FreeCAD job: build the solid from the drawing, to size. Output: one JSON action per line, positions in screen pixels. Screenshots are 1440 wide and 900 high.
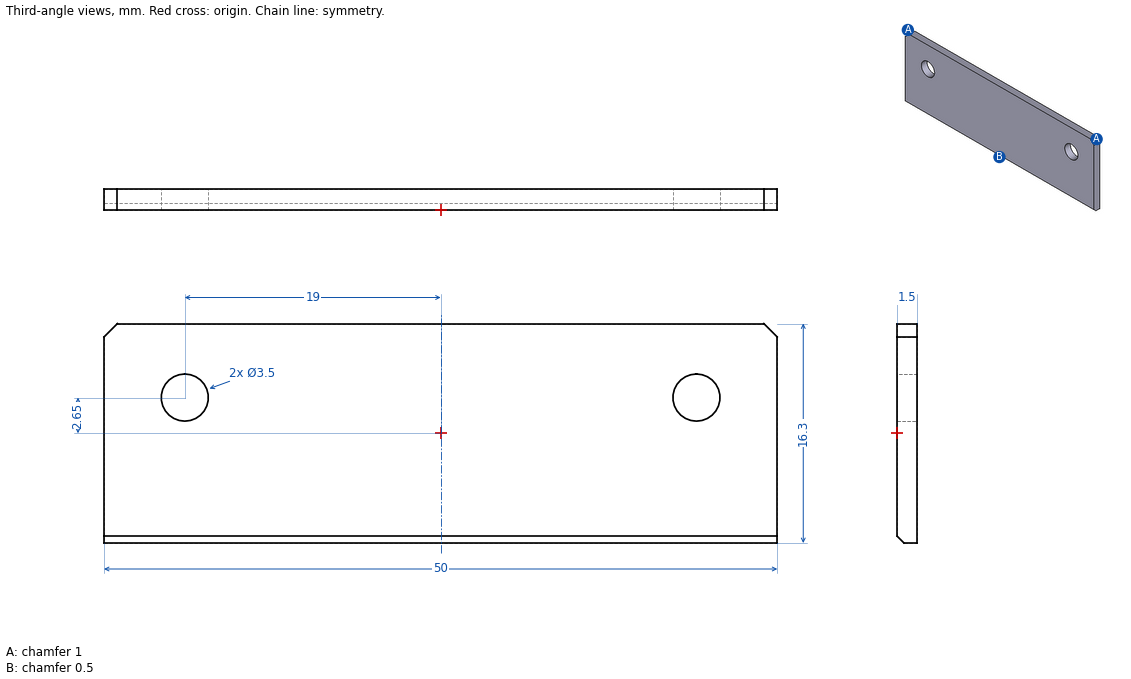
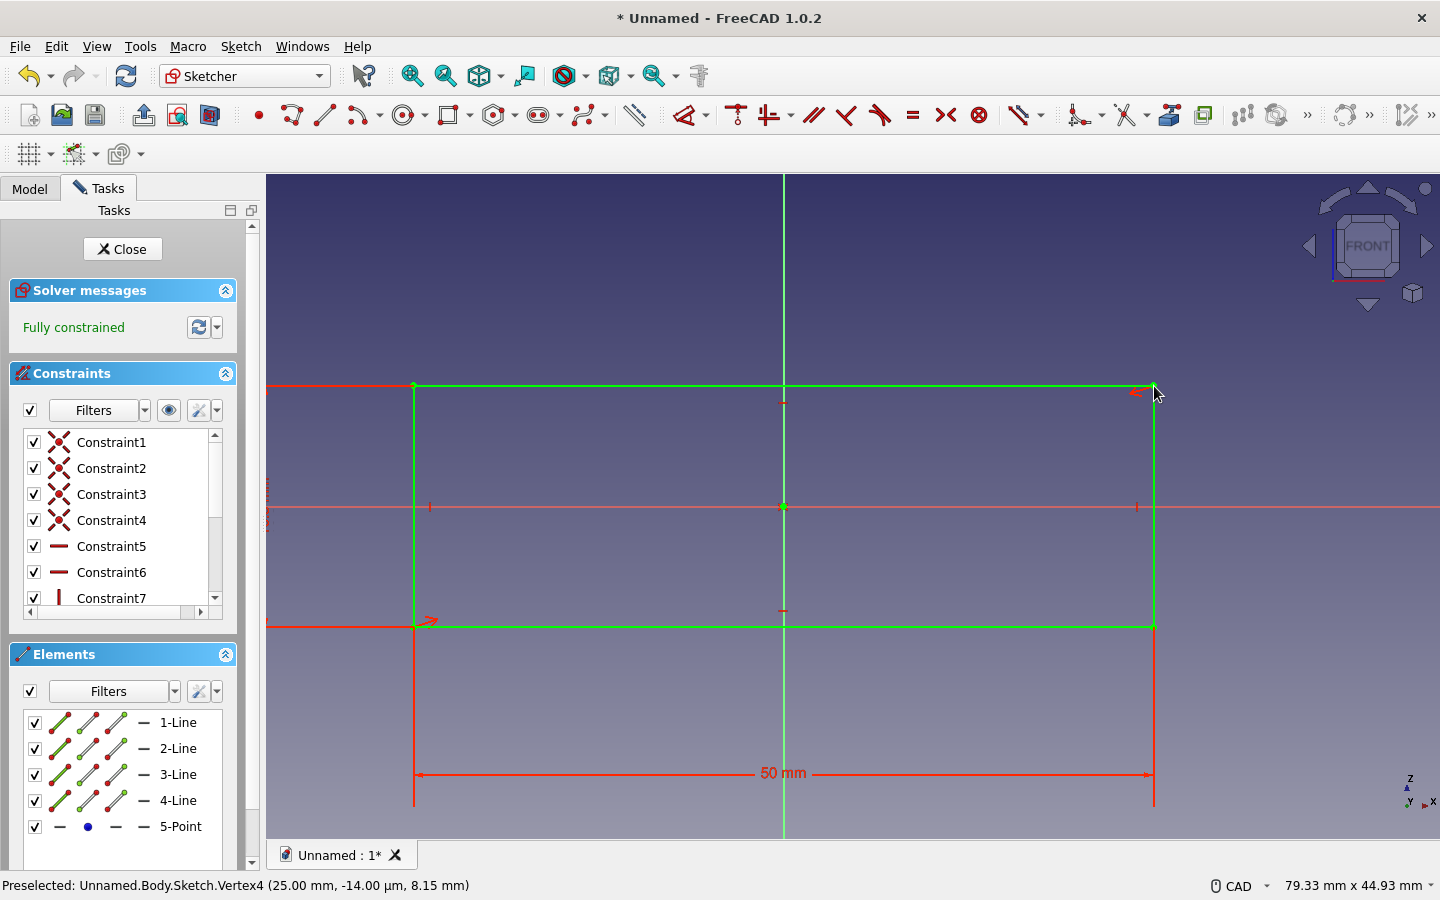
{"action": "left_click", "coordinate": [123, 249]}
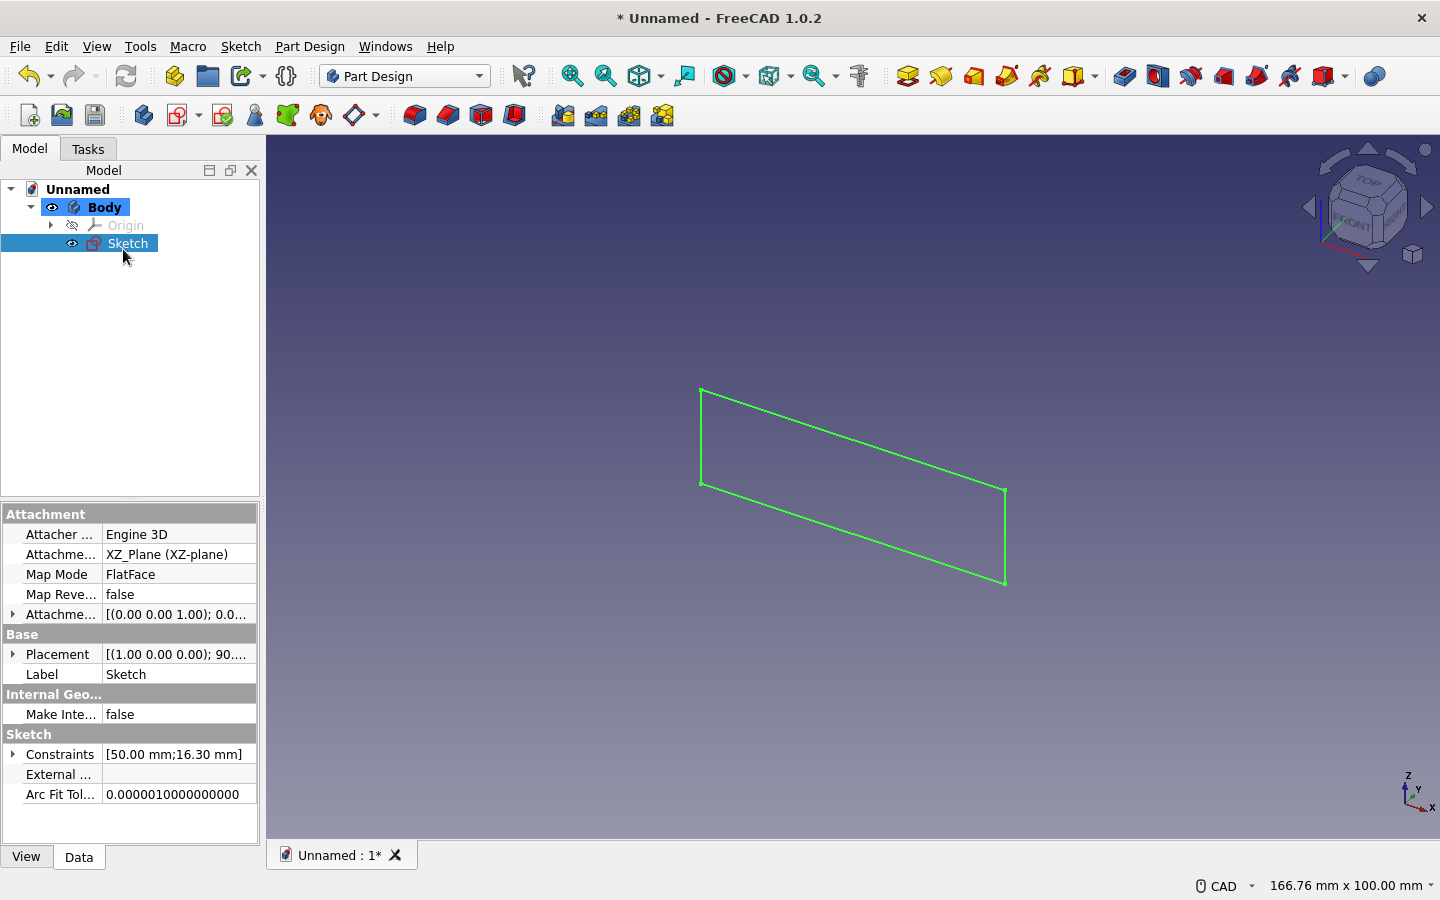
{"action": "left_click", "coordinate": [908, 76]}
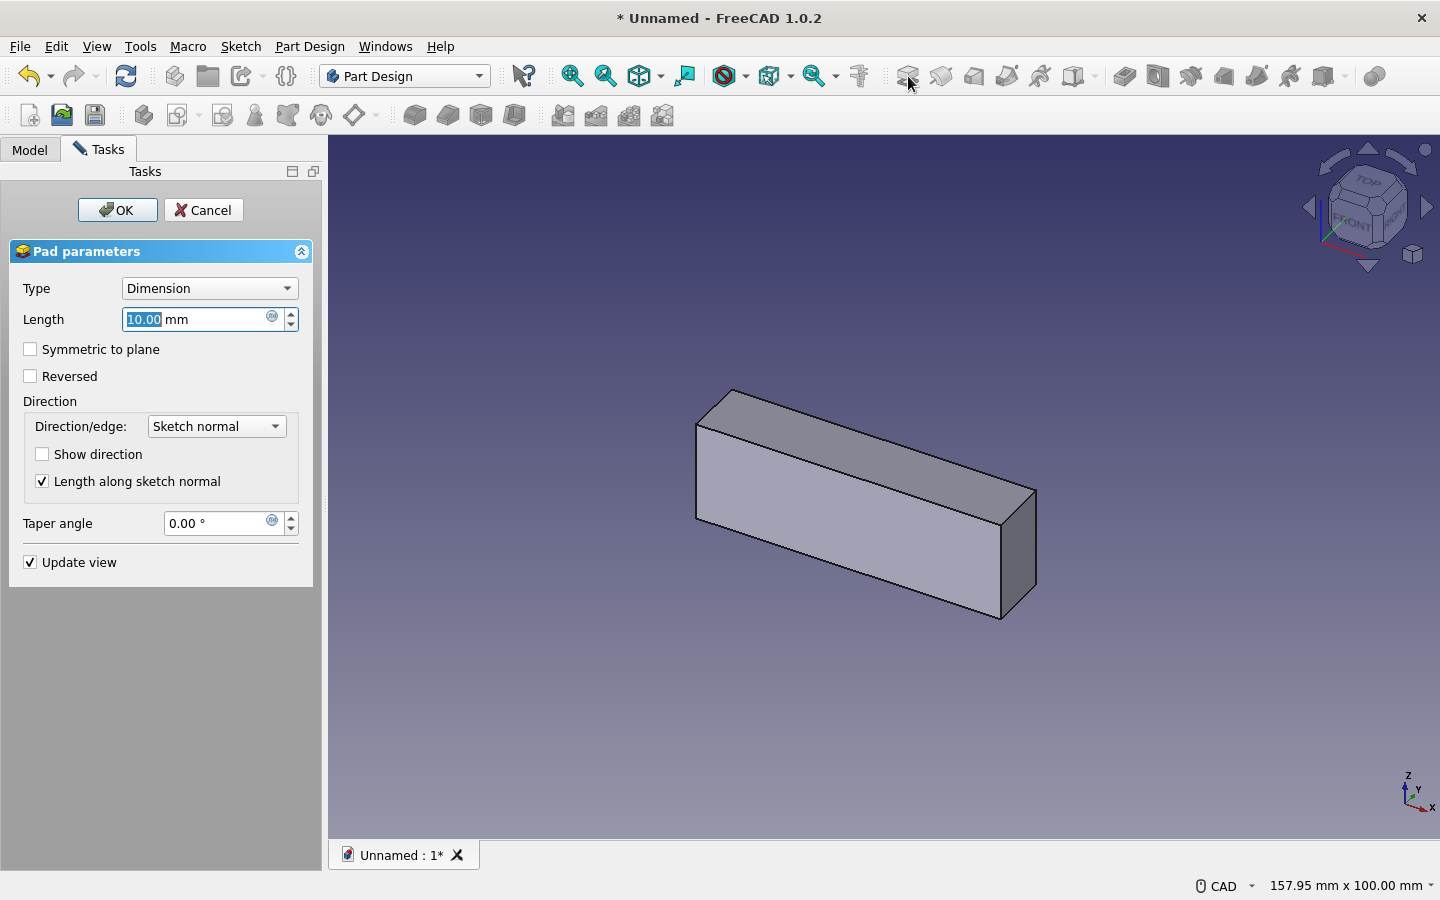
{"action": "type", "text": "1.5"}
{"action": "key", "text": "Tab"}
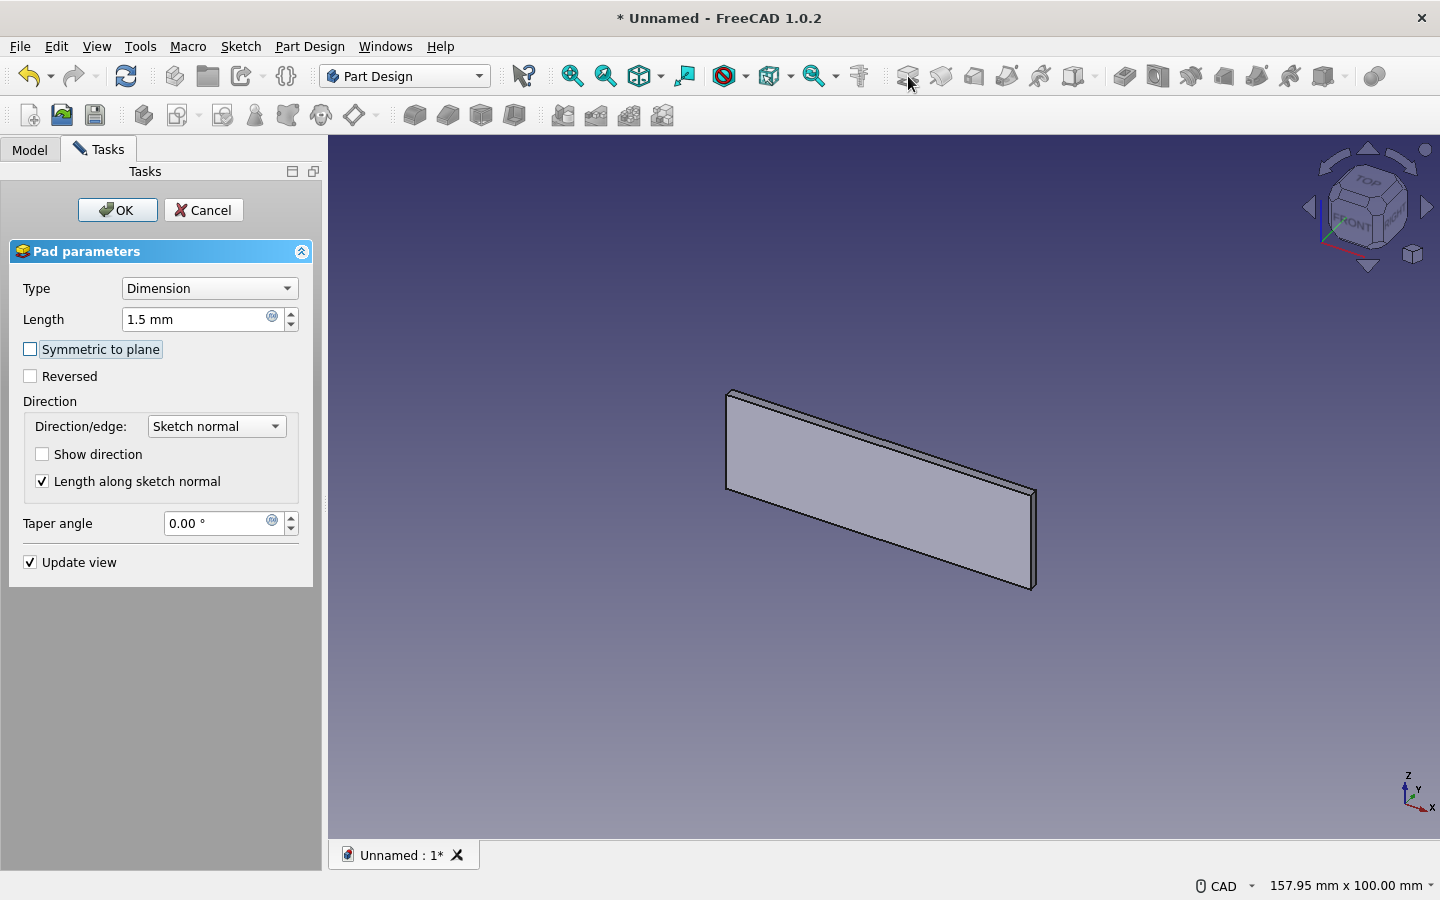
{"action": "left_click", "coordinate": [31, 376]}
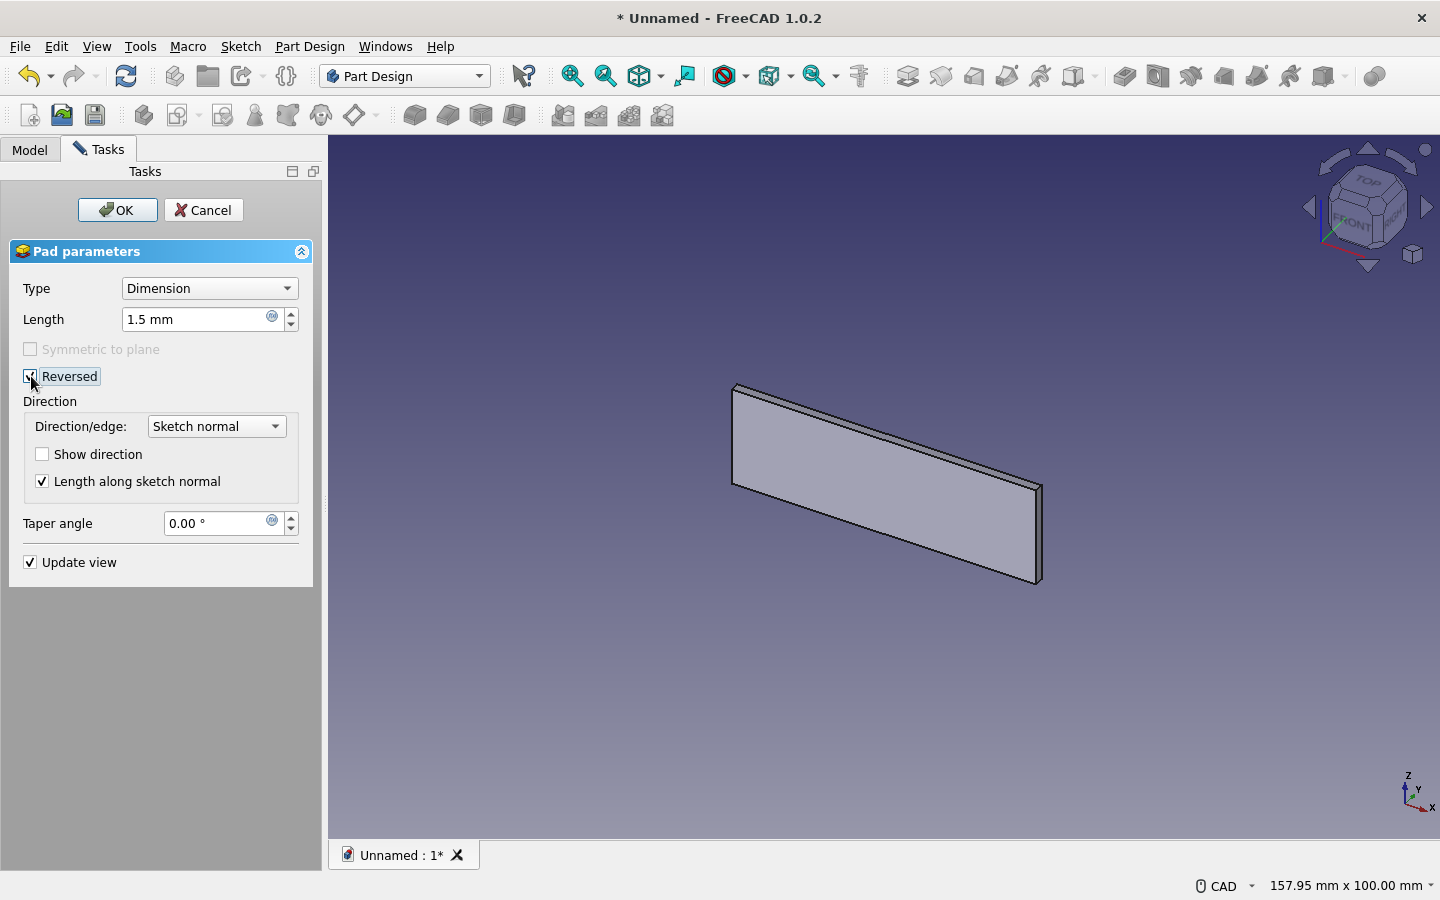
{"action": "left_click", "coordinate": [118, 210]}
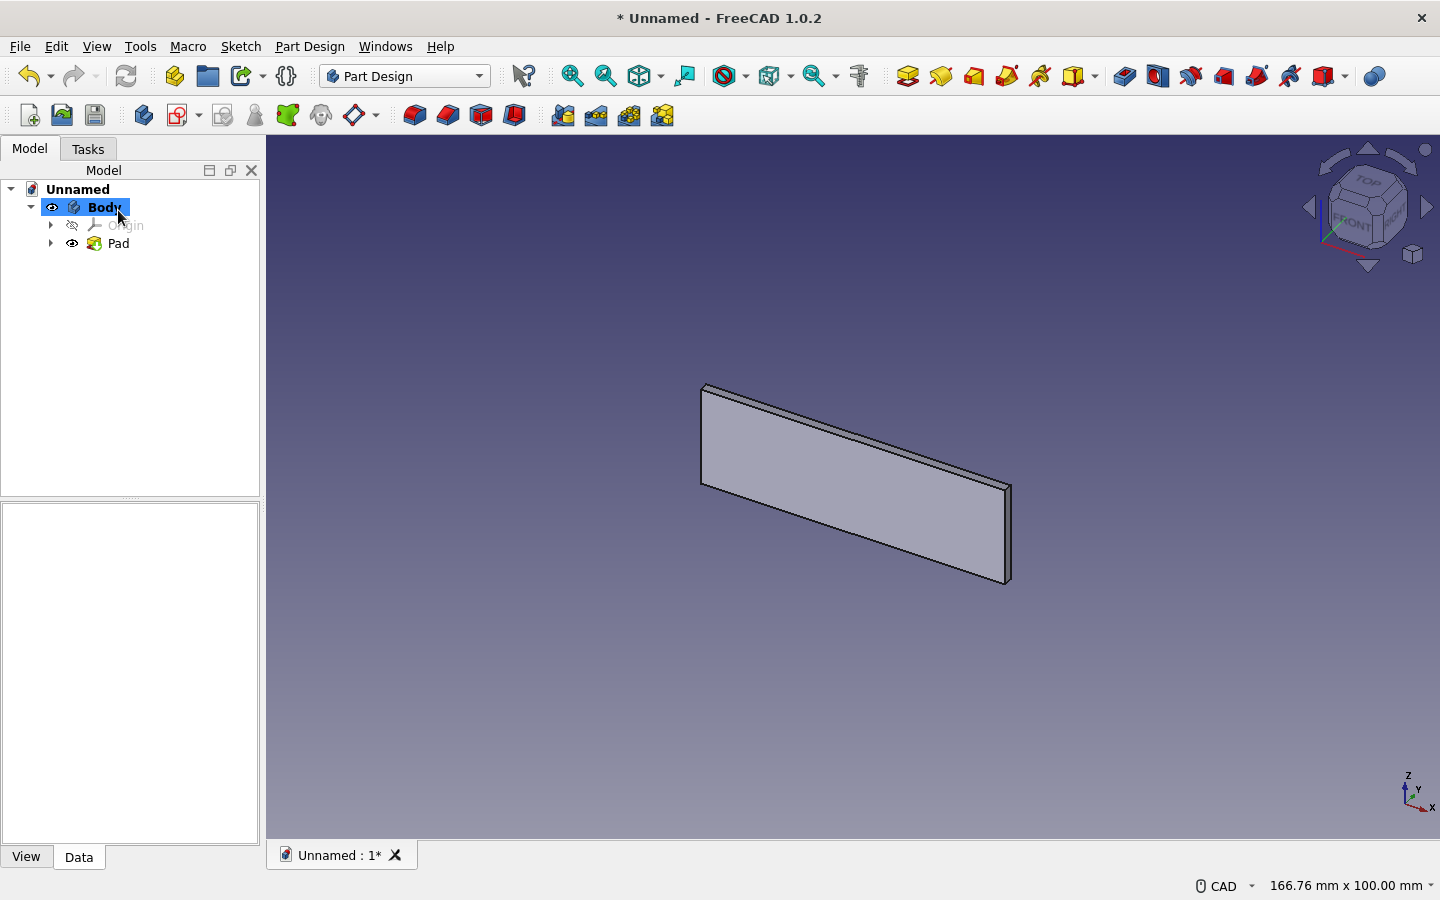
{"action": "key", "text": "v f"}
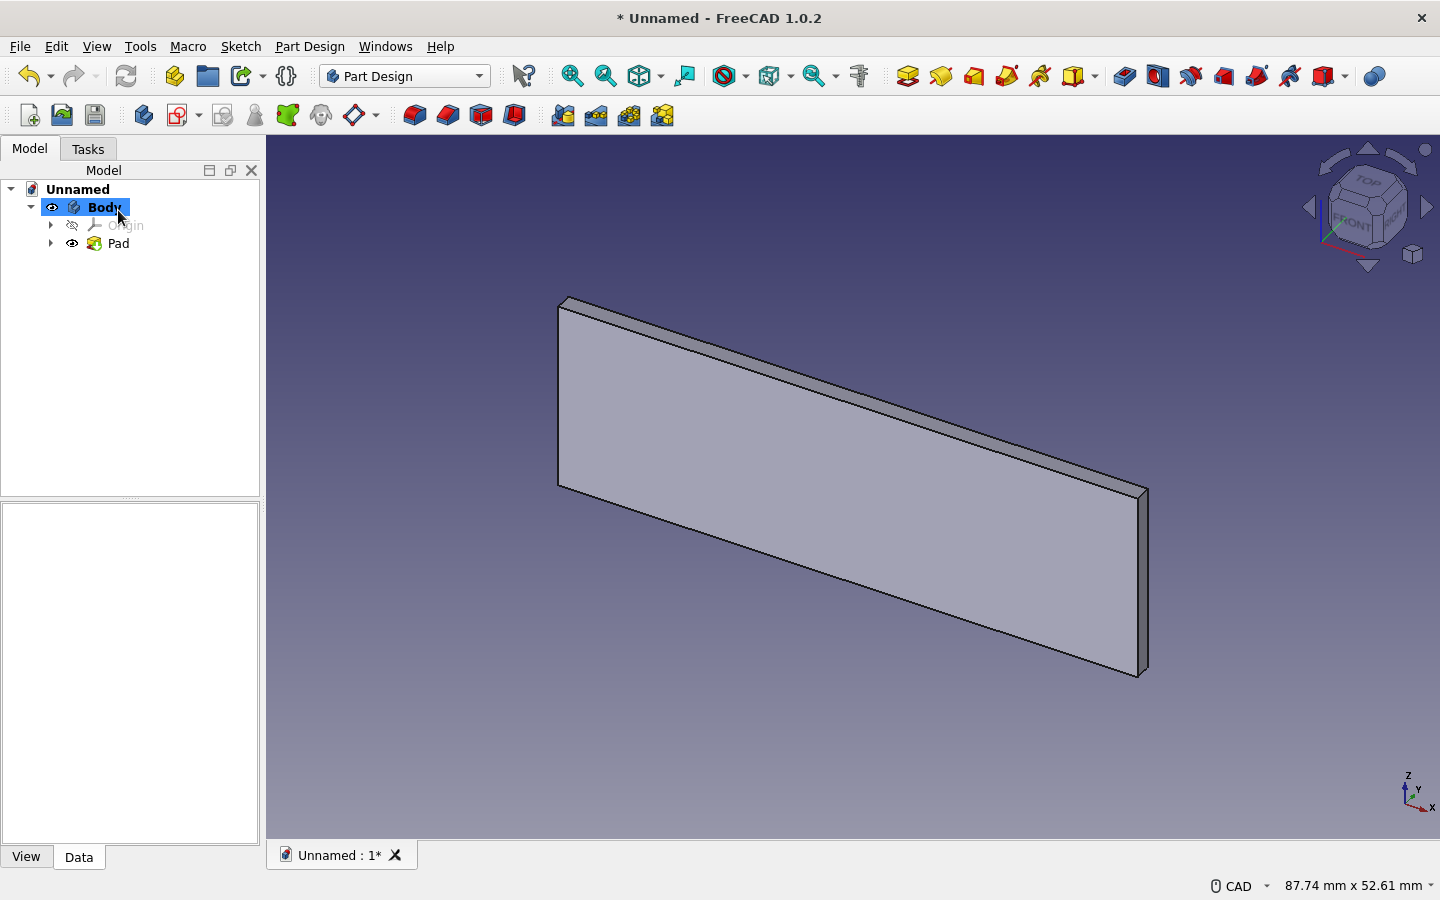
{"action": "key", "text": "4"}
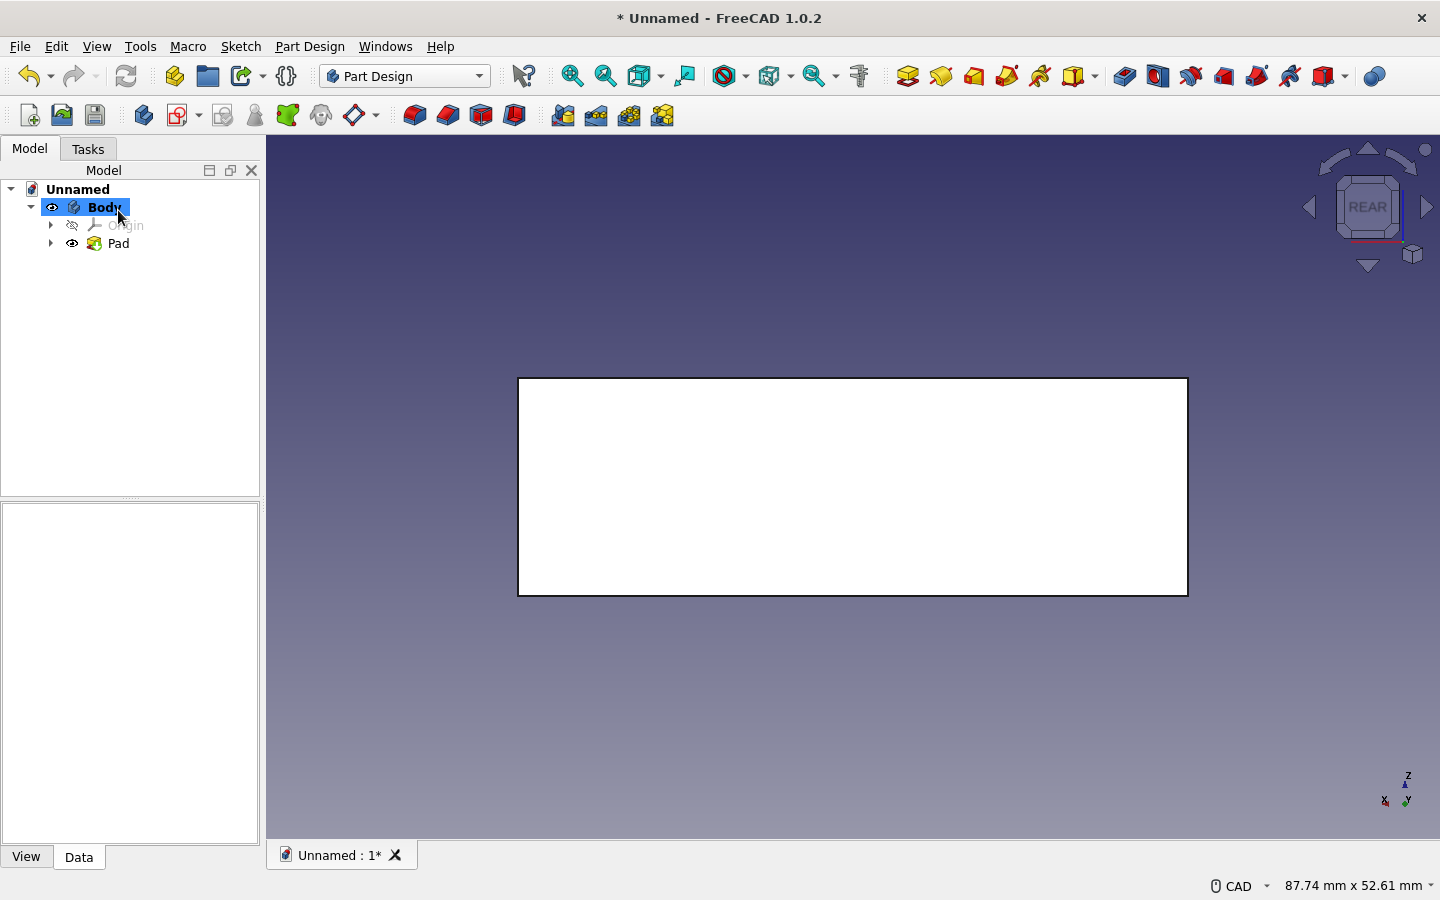
{"action": "left_click", "coordinate": [662, 486]}